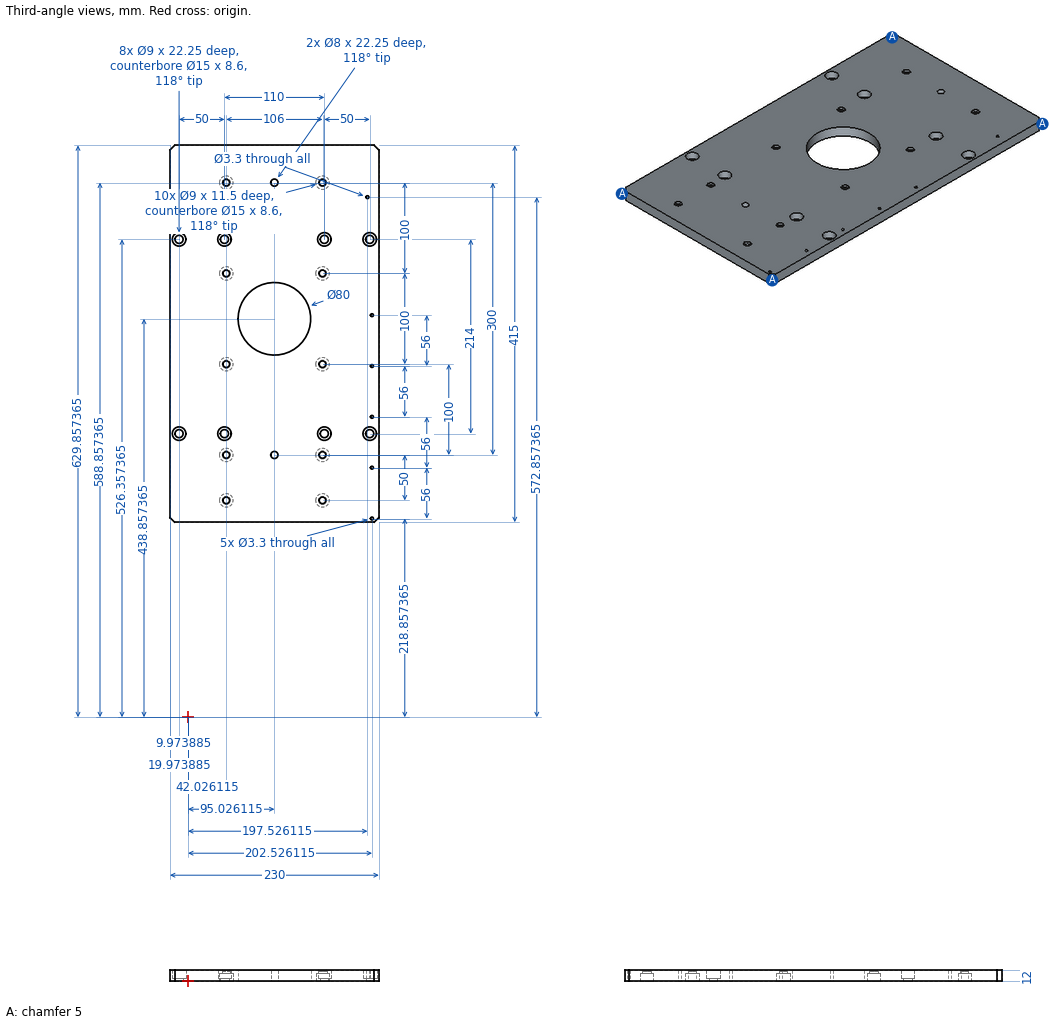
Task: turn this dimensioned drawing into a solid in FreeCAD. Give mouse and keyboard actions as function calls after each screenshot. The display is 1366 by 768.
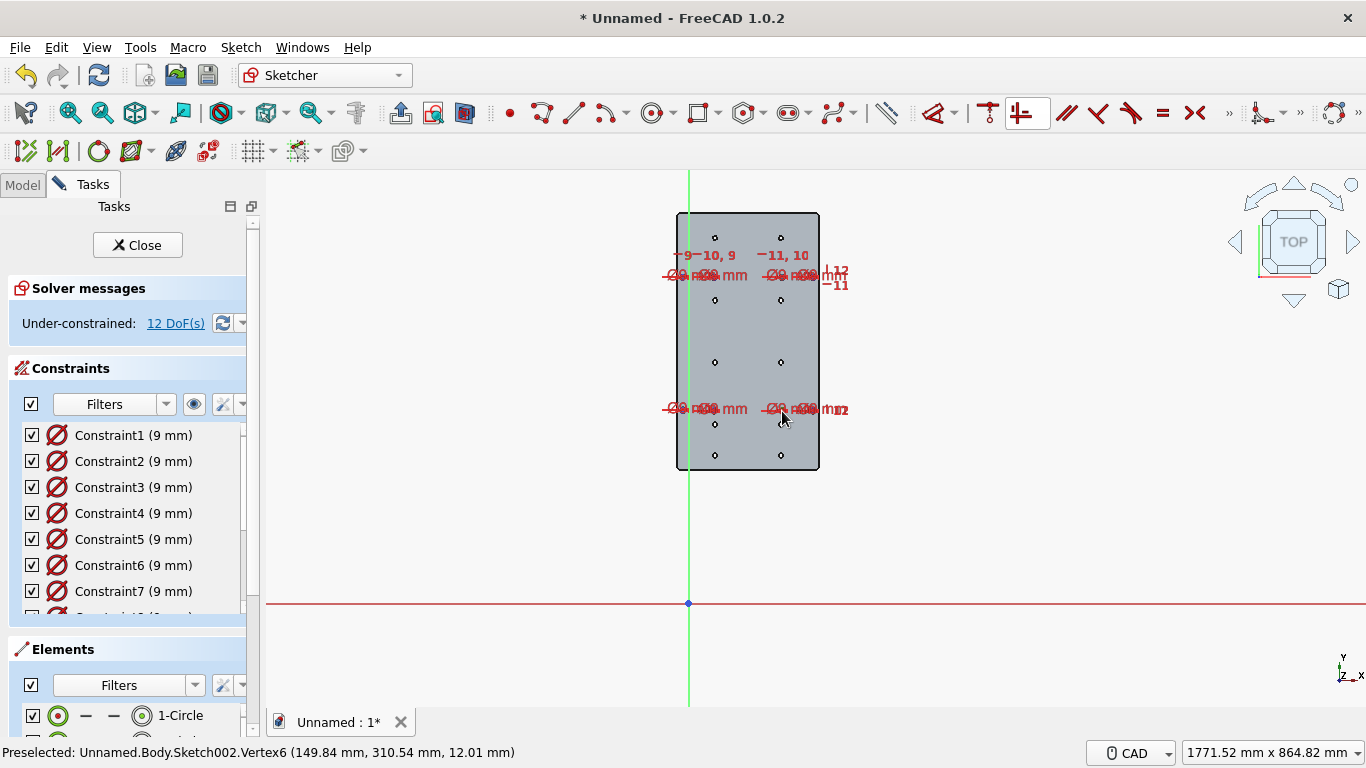
key(v)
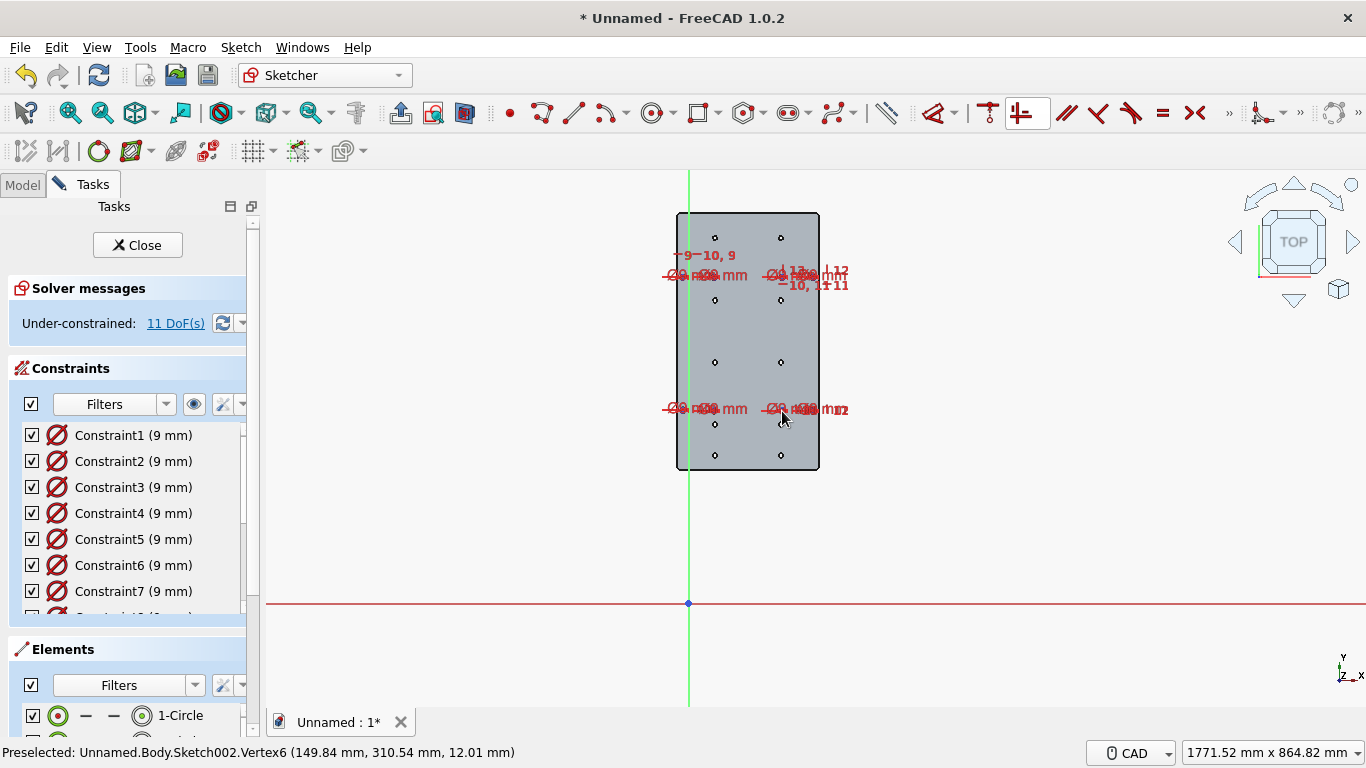
scroll(813, 411, up, 4)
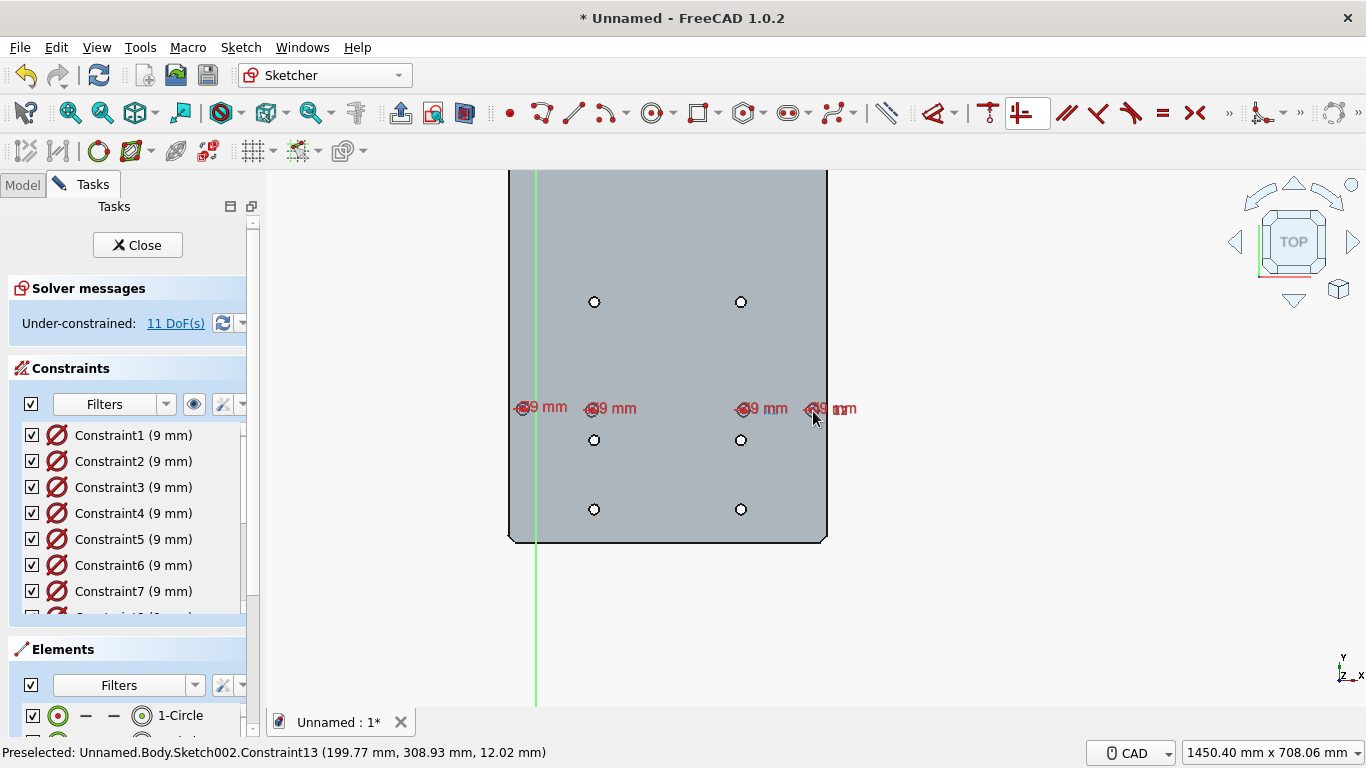
click(812, 410)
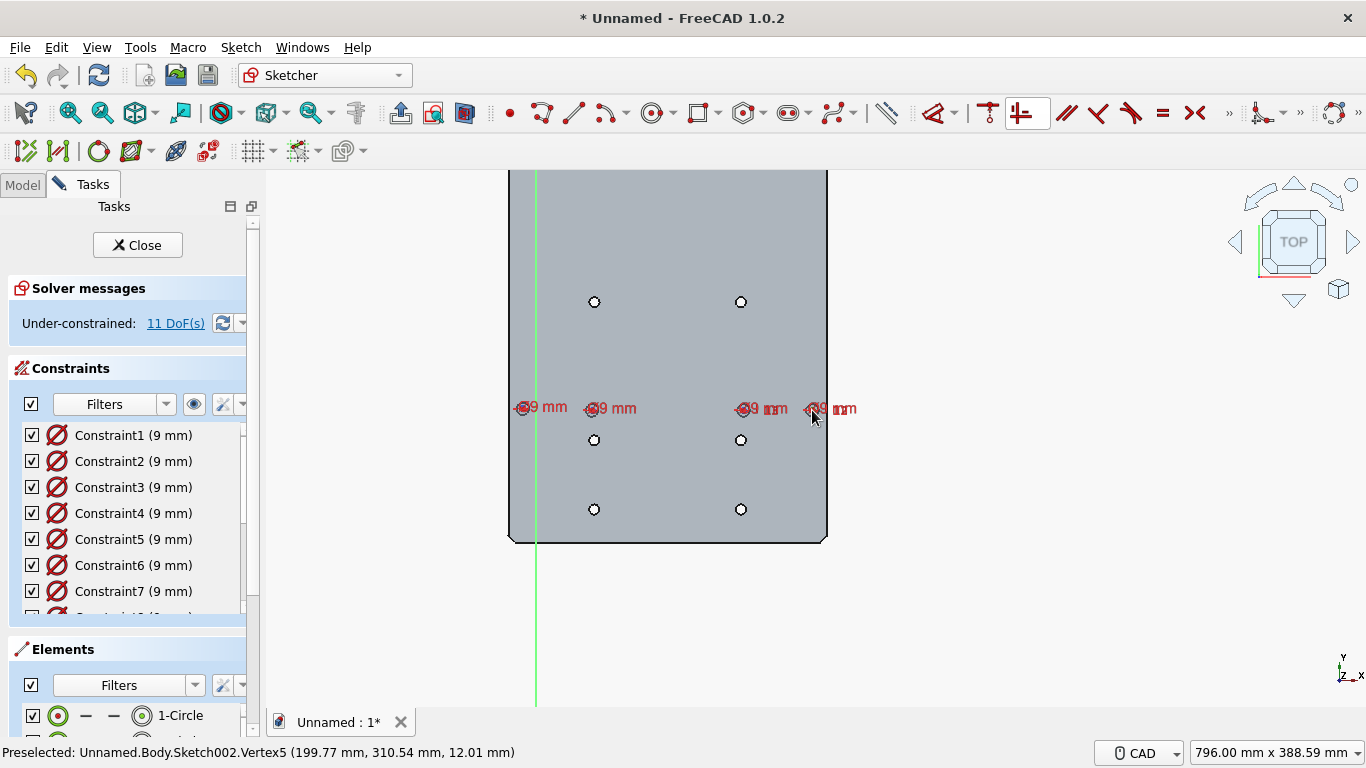
click(743, 410)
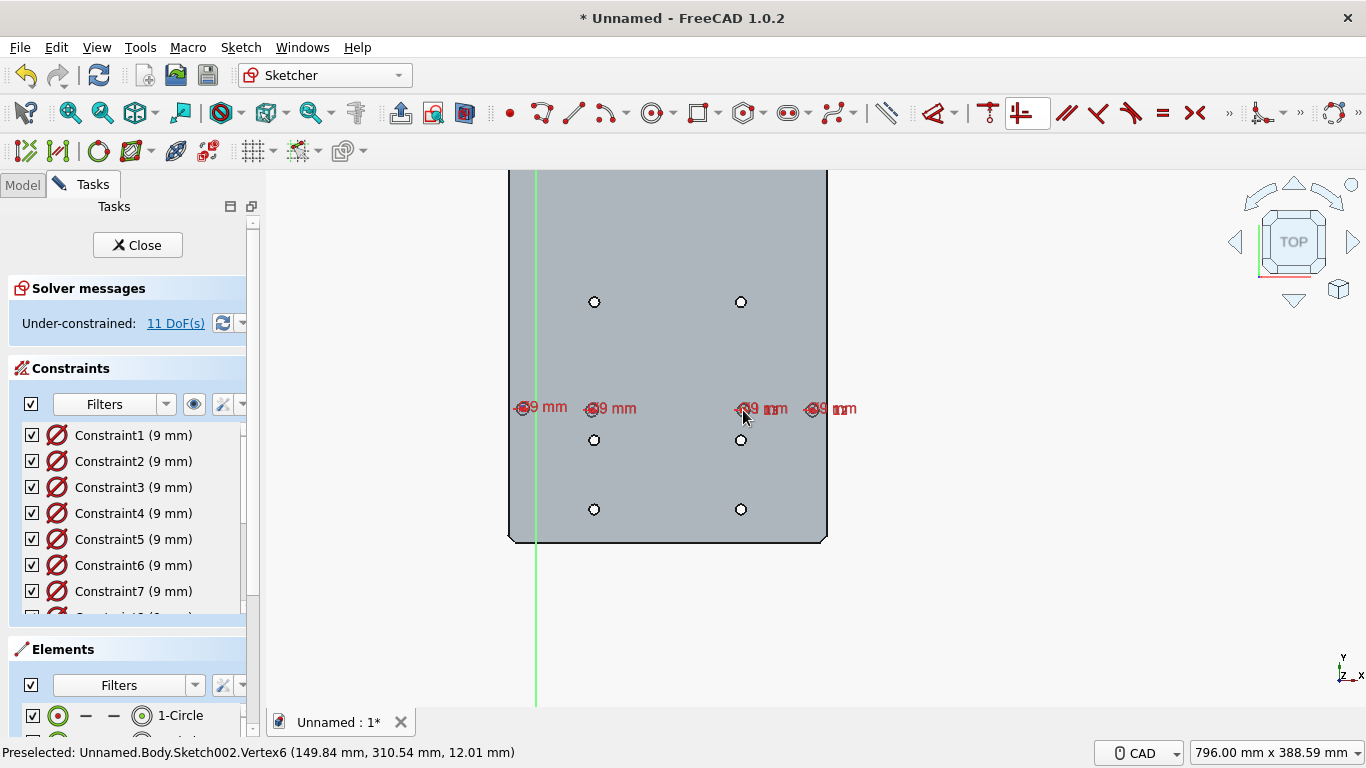
key(h)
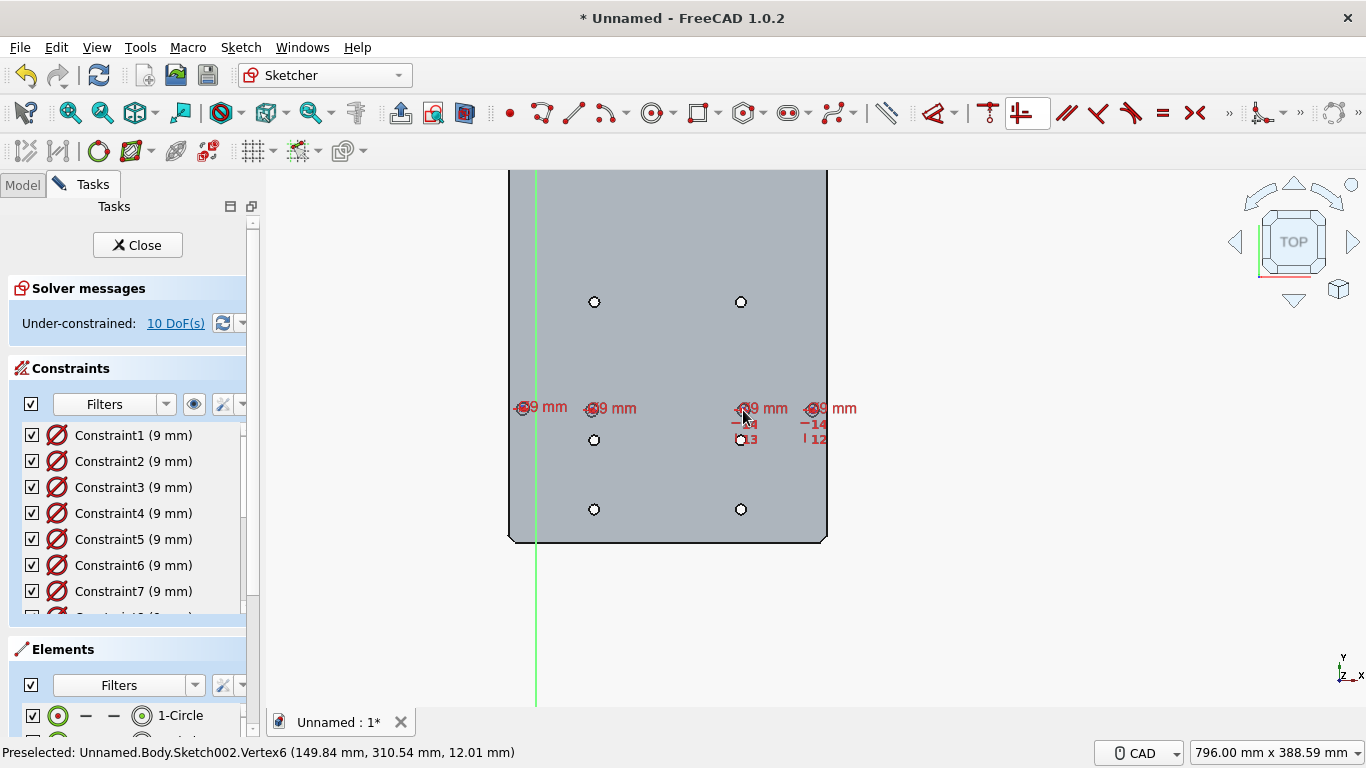
scroll(813, 411, down, 4)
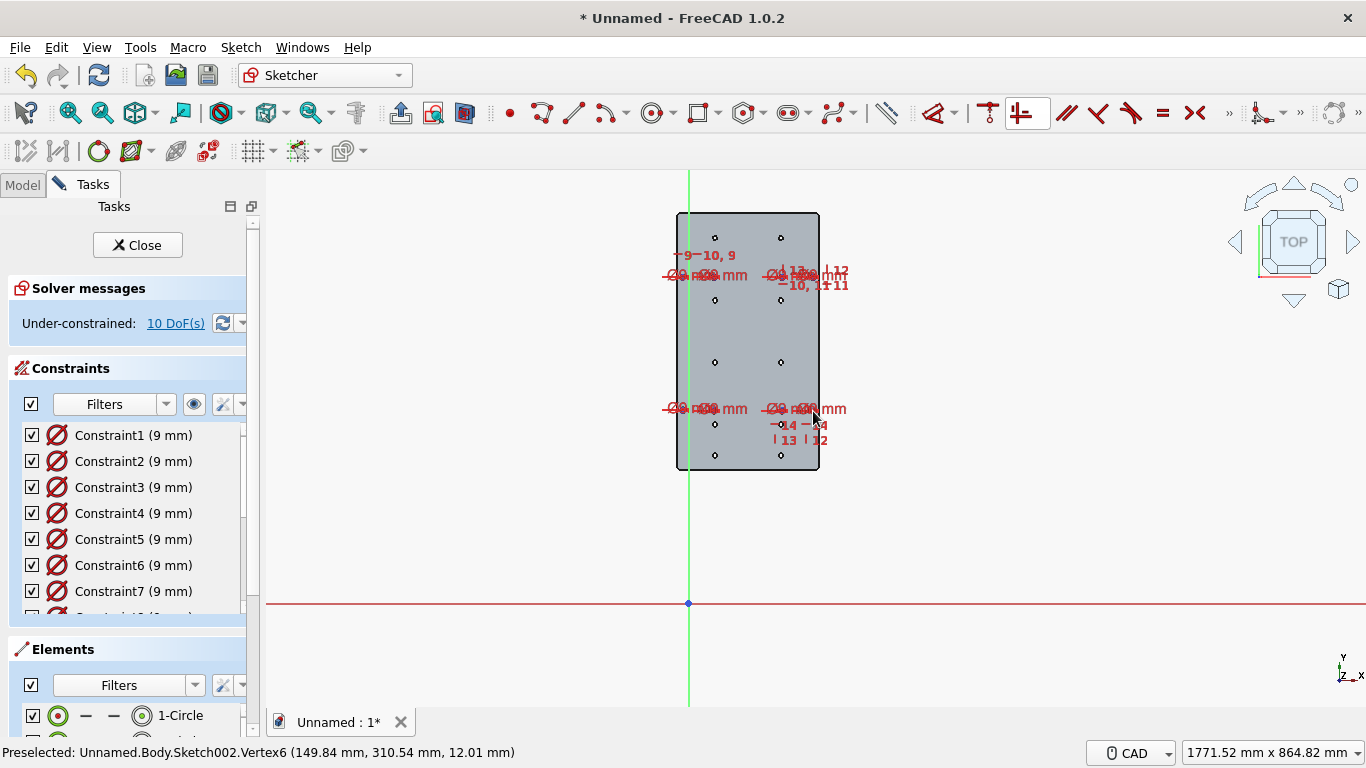
click(714, 277)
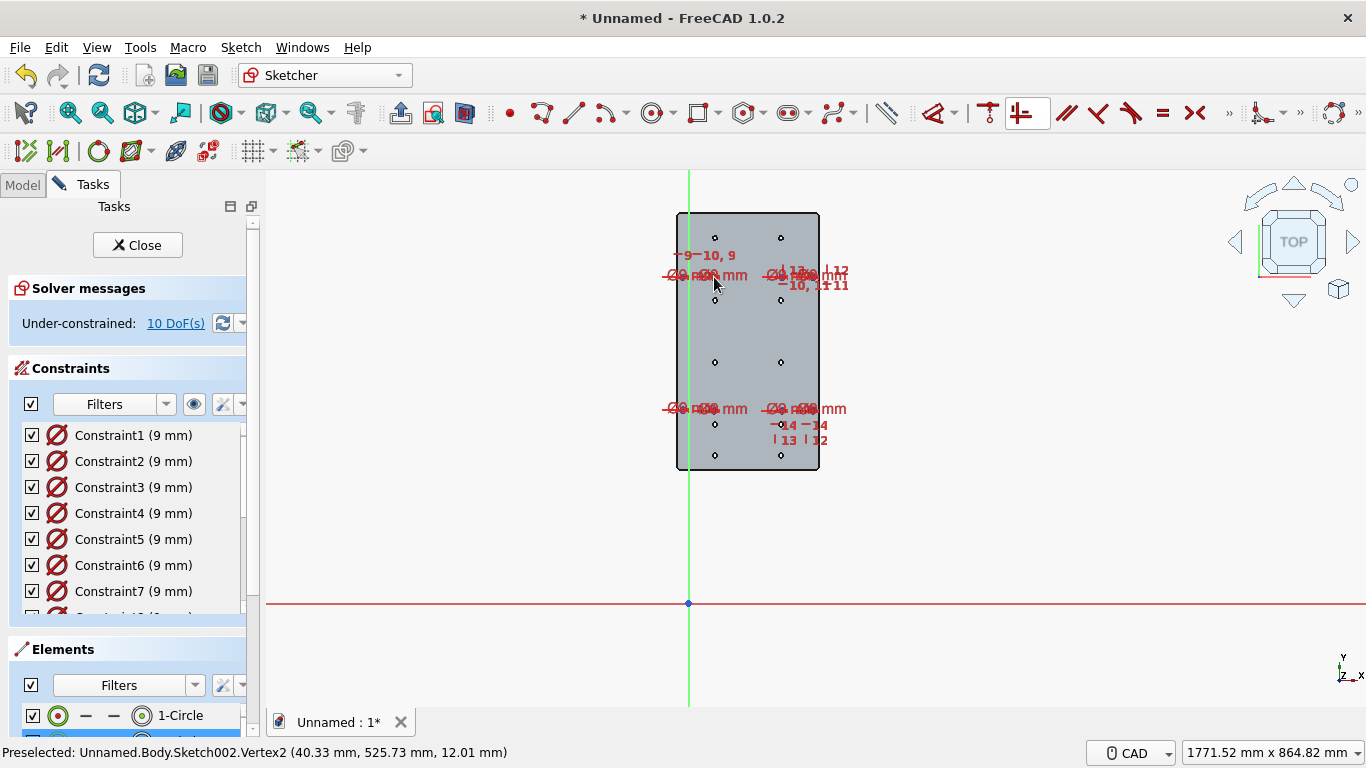
click(714, 411)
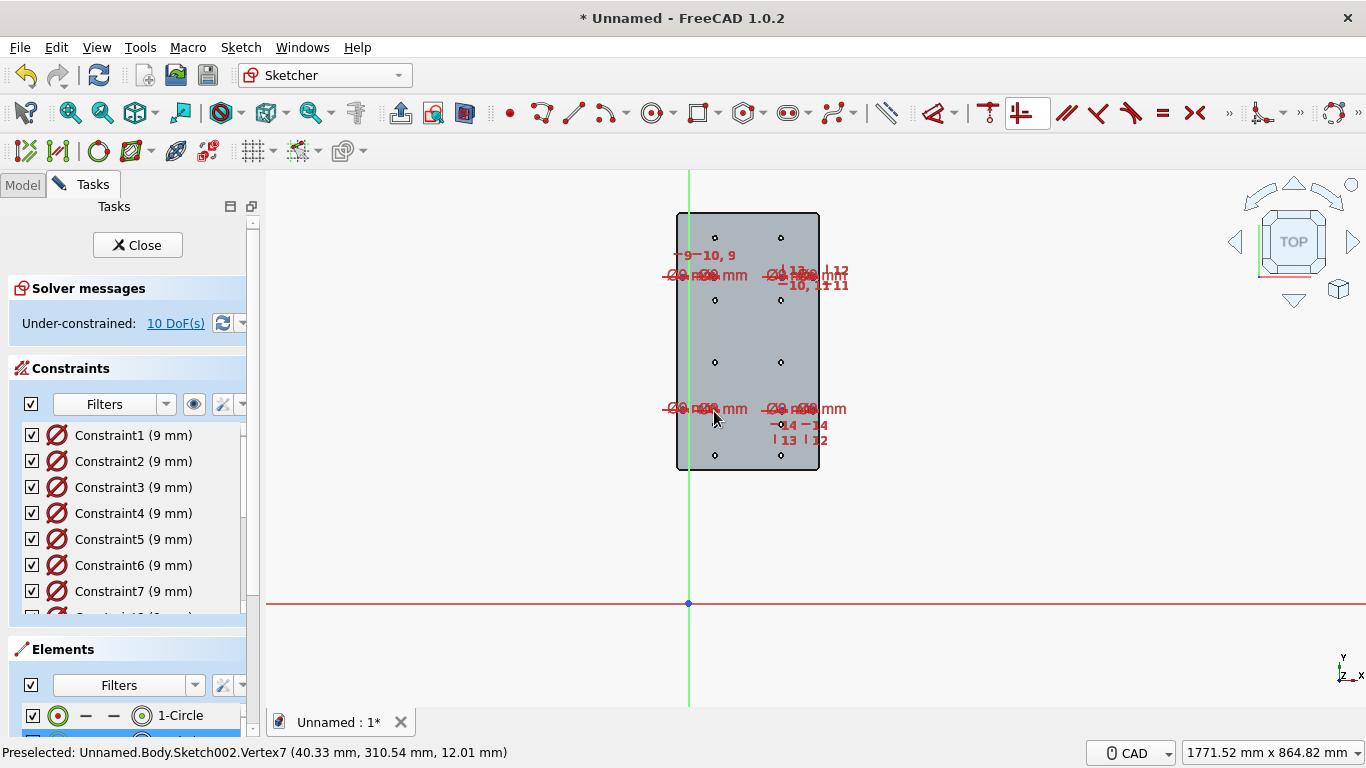
click(1044, 114)